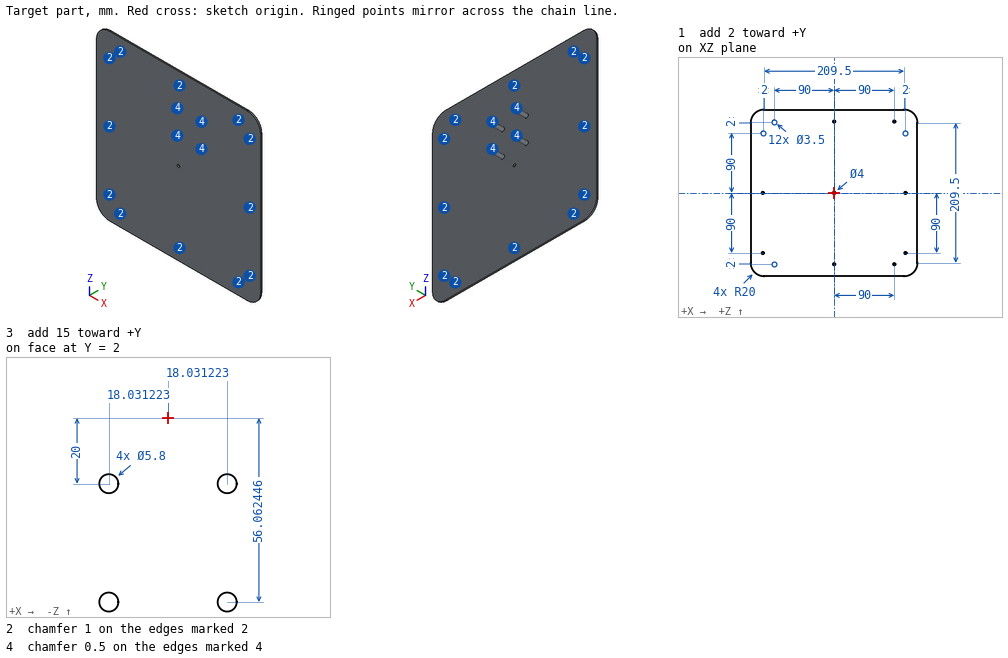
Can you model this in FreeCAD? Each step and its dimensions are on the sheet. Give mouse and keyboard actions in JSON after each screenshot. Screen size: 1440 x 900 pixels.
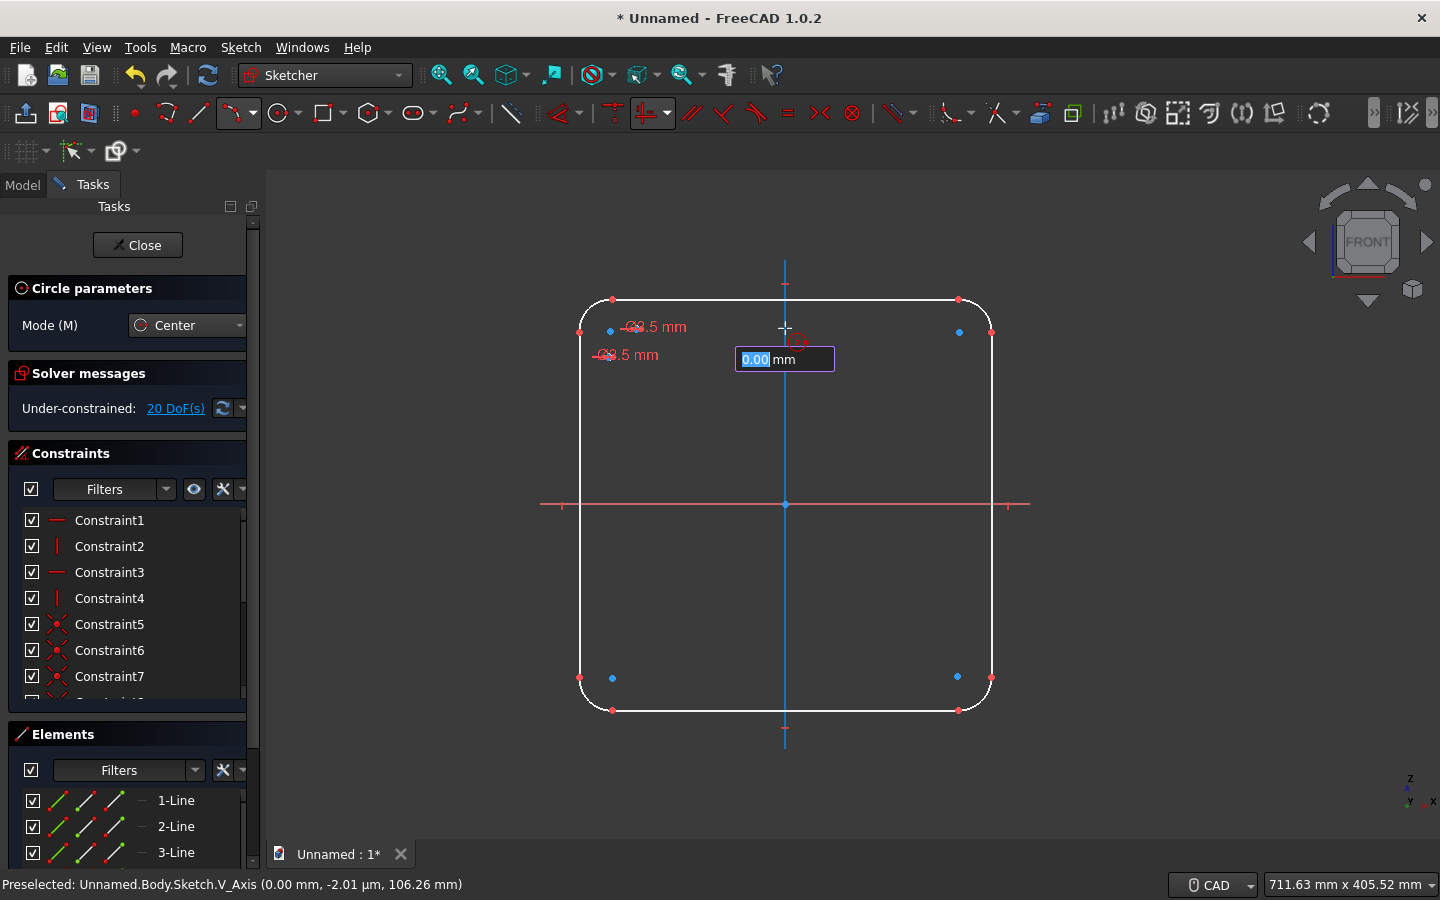
{"action": "scroll", "coordinate": [788, 327], "scroll_direction": "up", "scroll_amount": 9}
{"action": "mouse_move", "coordinate": [786, 327]}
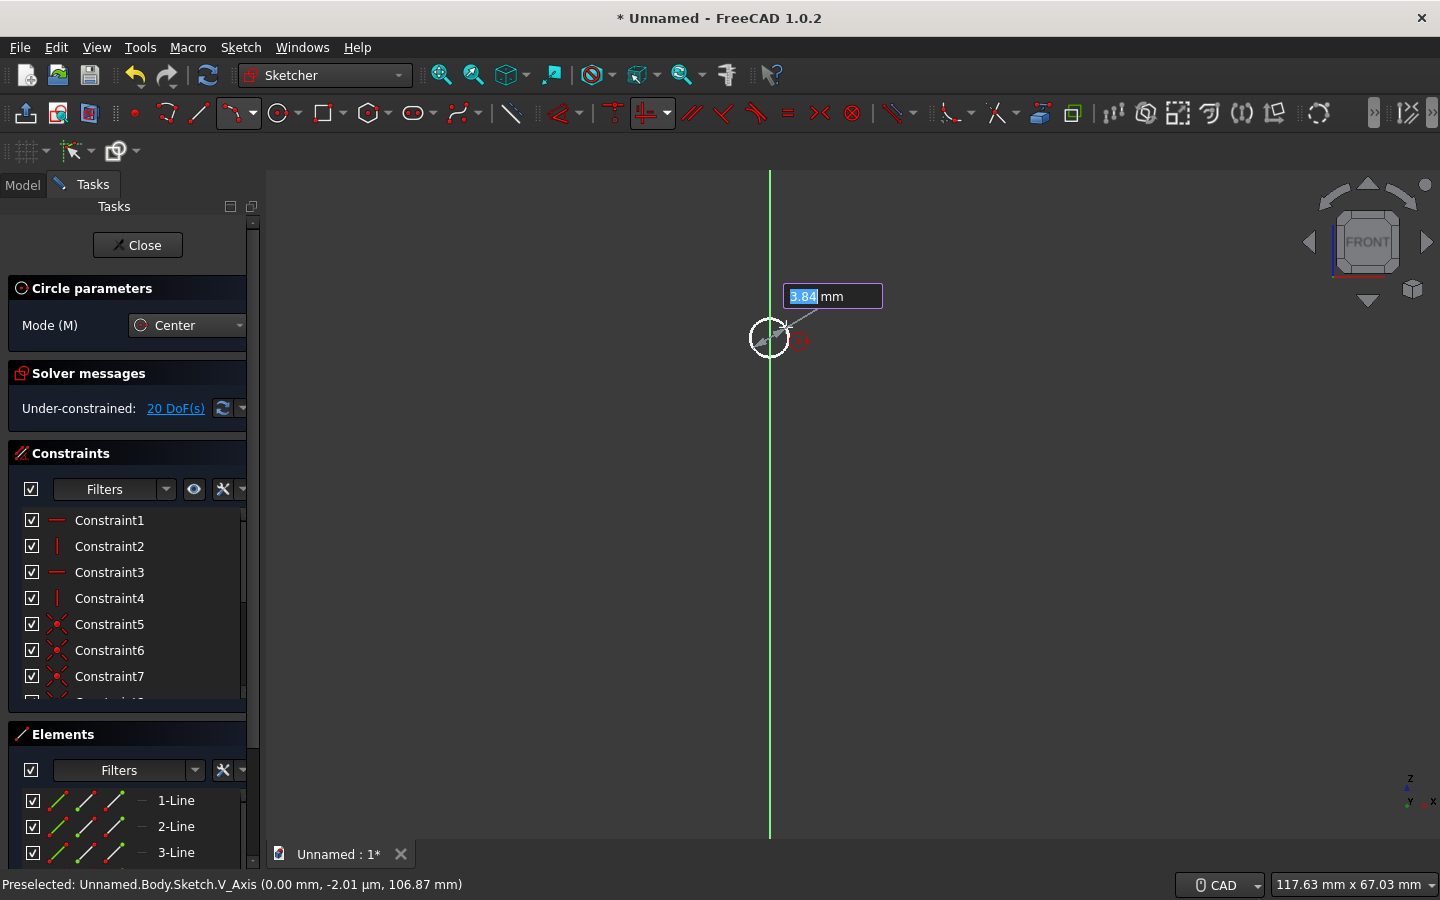
{"action": "type", "text": "3.5"}
{"action": "key", "text": "Return"}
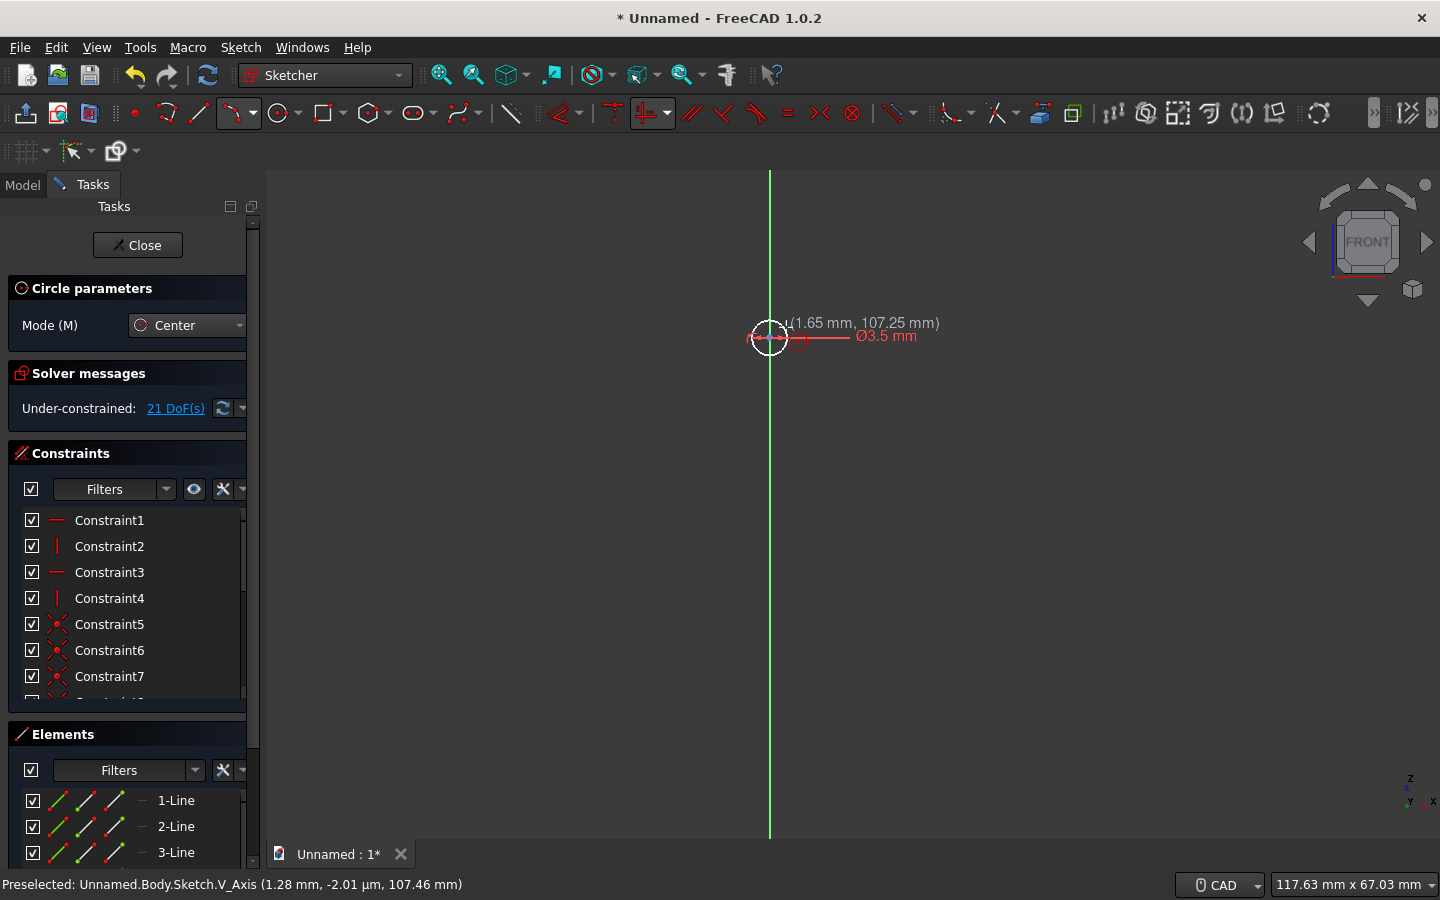
{"action": "scroll", "coordinate": [787, 327], "scroll_direction": "down", "scroll_amount": 9}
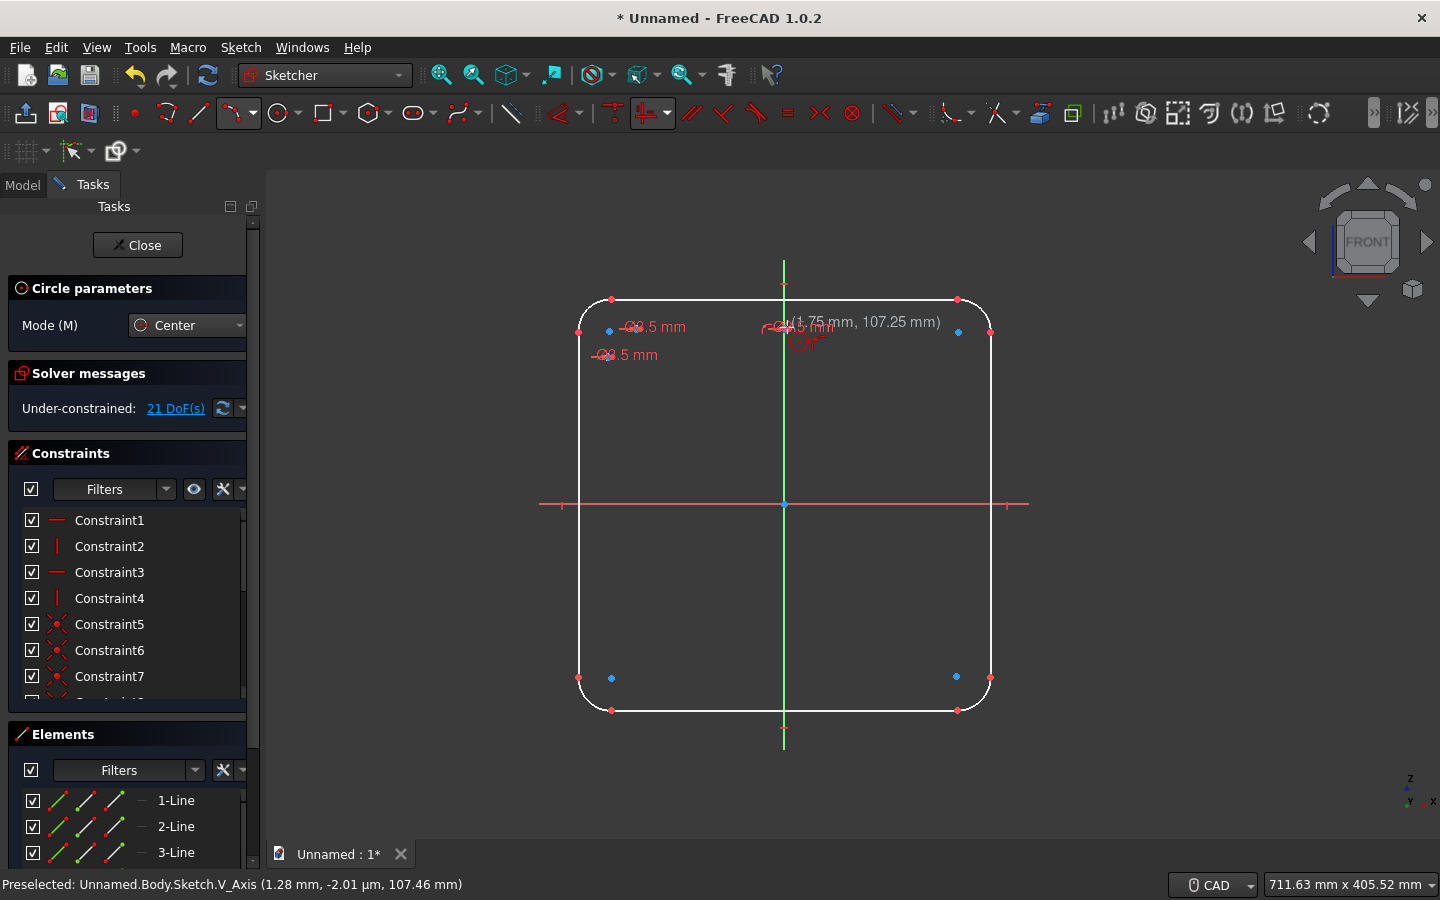
{"action": "scroll", "coordinate": [933, 328], "scroll_direction": "up", "scroll_amount": 11}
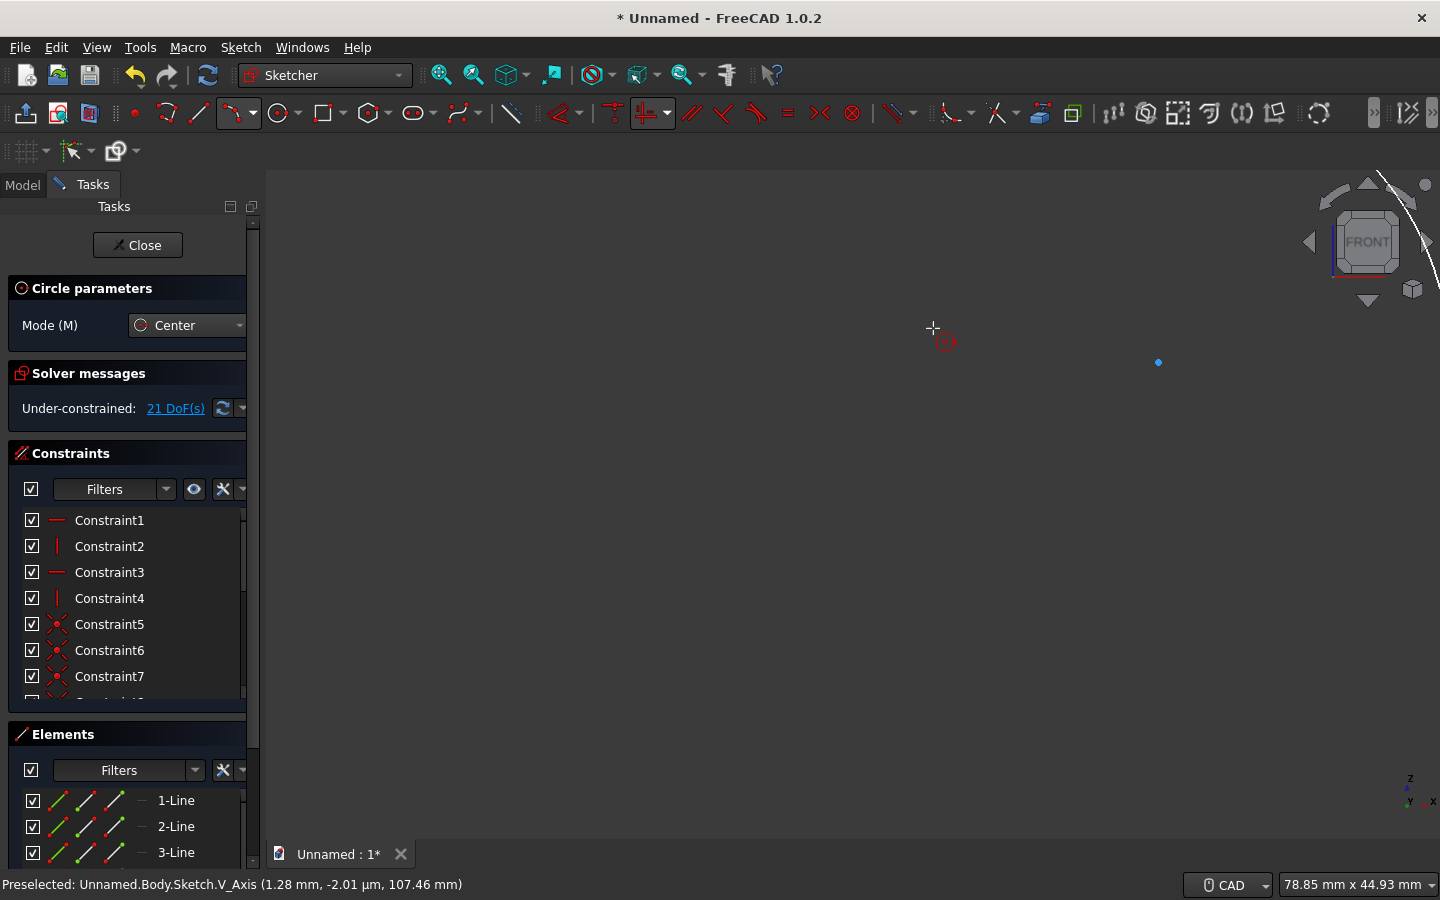
{"action": "scroll", "coordinate": [934, 328], "scroll_direction": "down", "scroll_amount": 11}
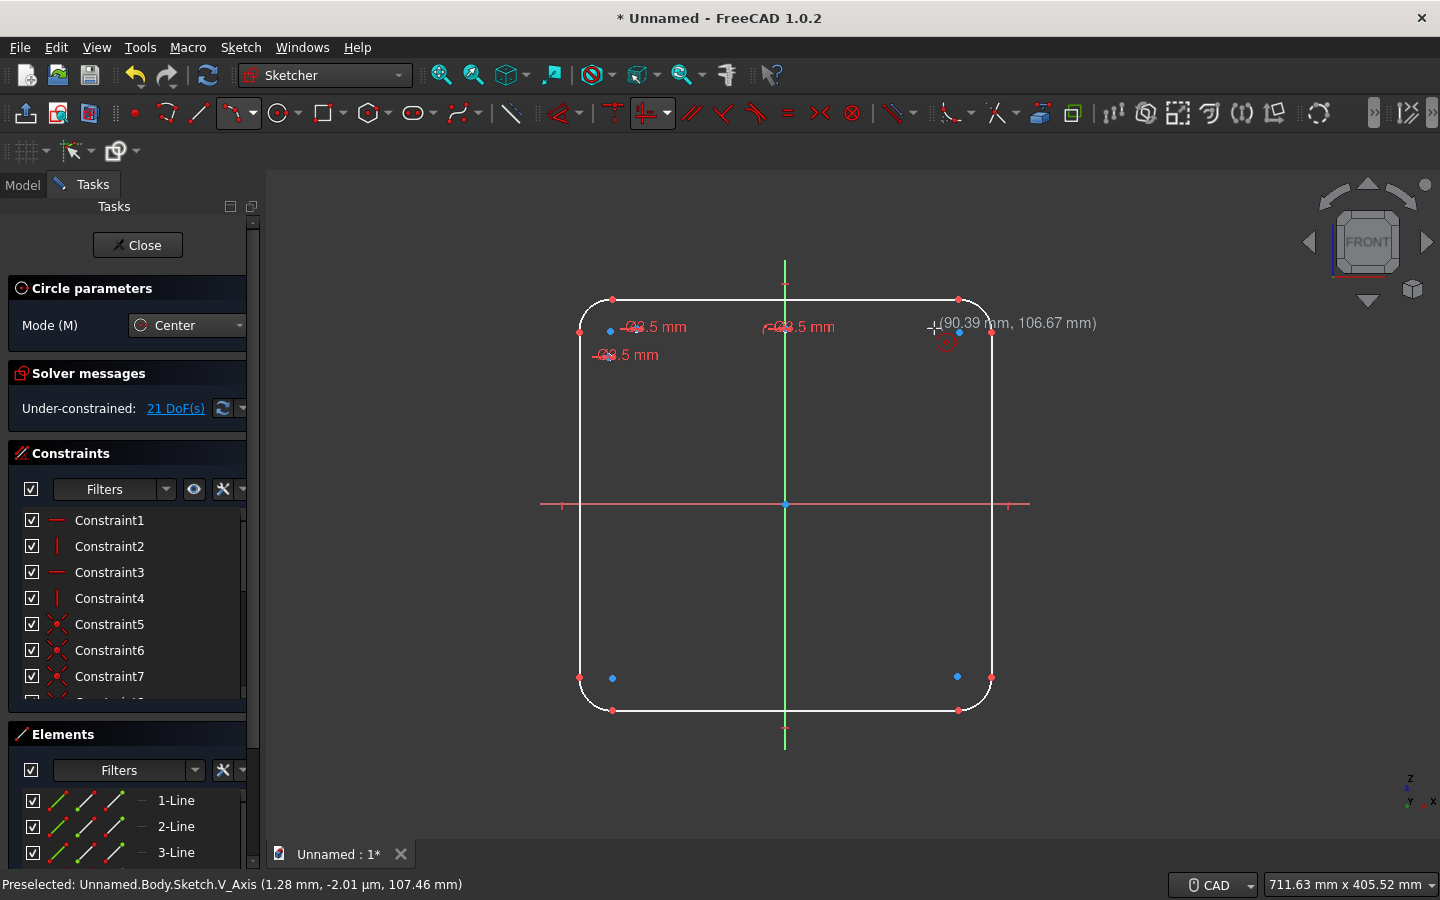
{"action": "left_click", "coordinate": [934, 328]}
{"action": "mouse_move", "coordinate": [936, 326]}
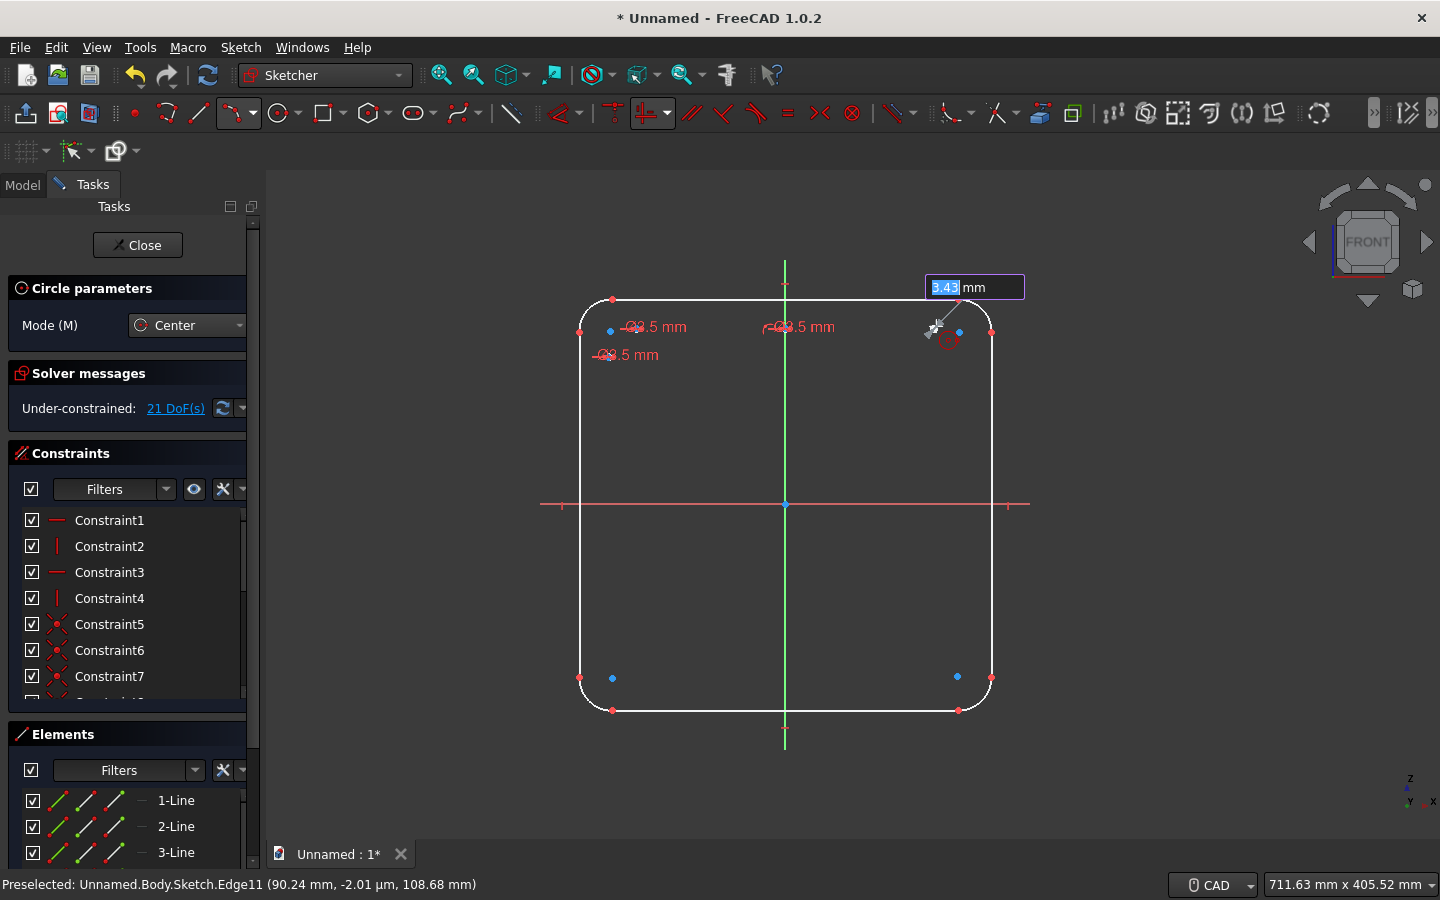
{"action": "type", "text": "3.5"}
{"action": "key", "text": "Return"}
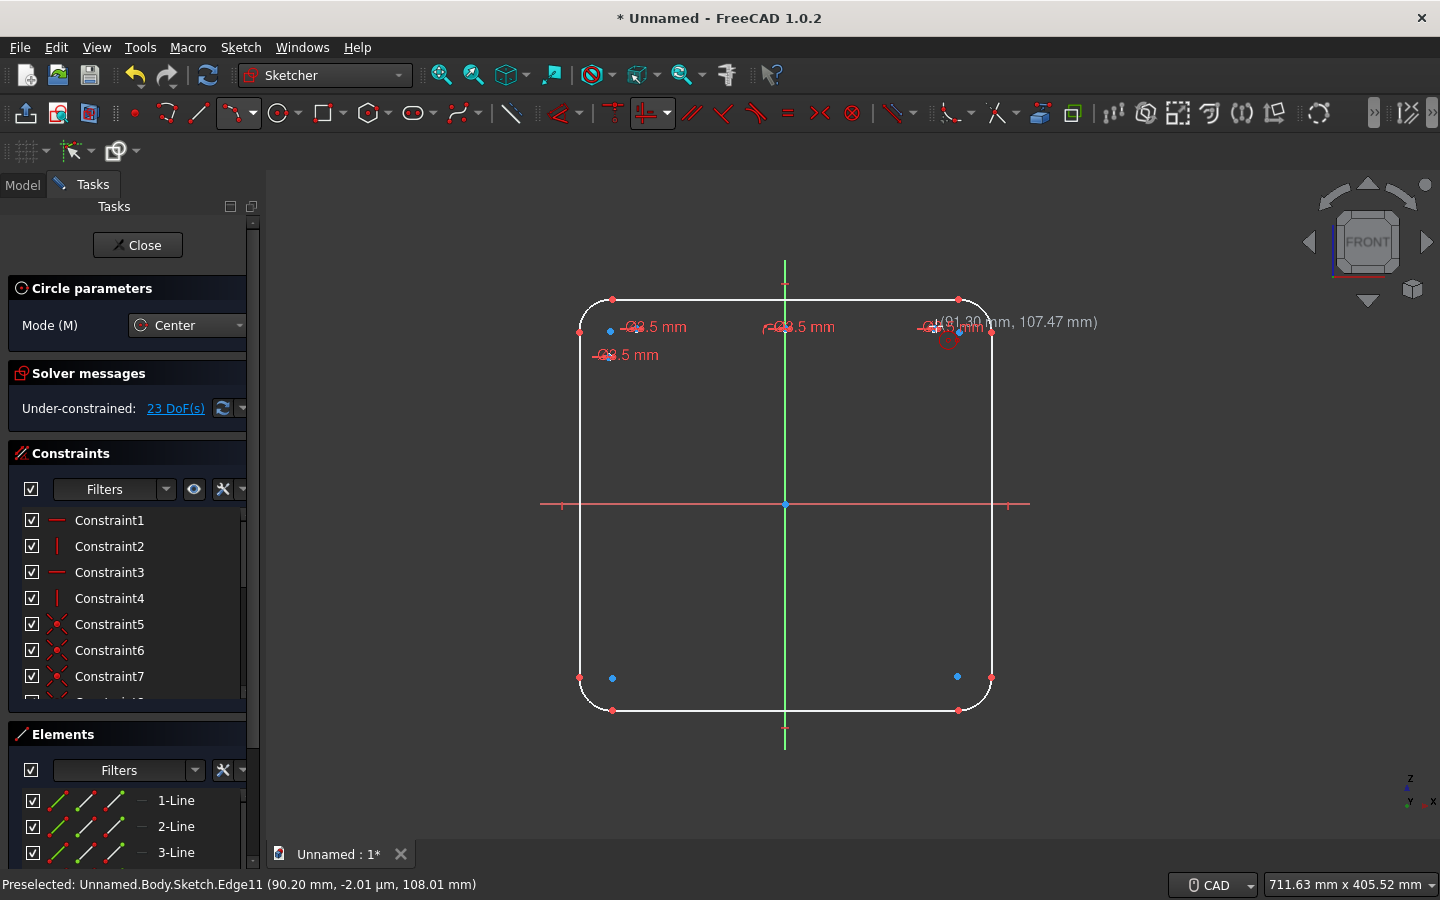
{"action": "scroll", "coordinate": [961, 356], "scroll_direction": "up", "scroll_amount": 11}